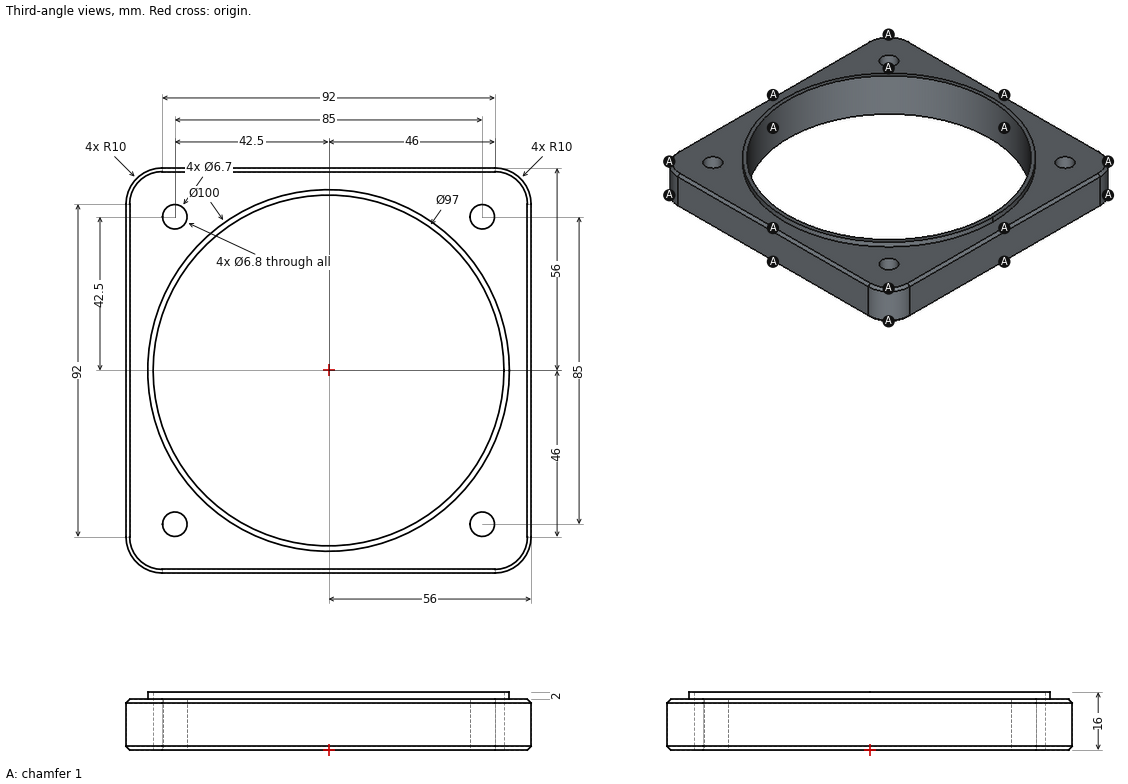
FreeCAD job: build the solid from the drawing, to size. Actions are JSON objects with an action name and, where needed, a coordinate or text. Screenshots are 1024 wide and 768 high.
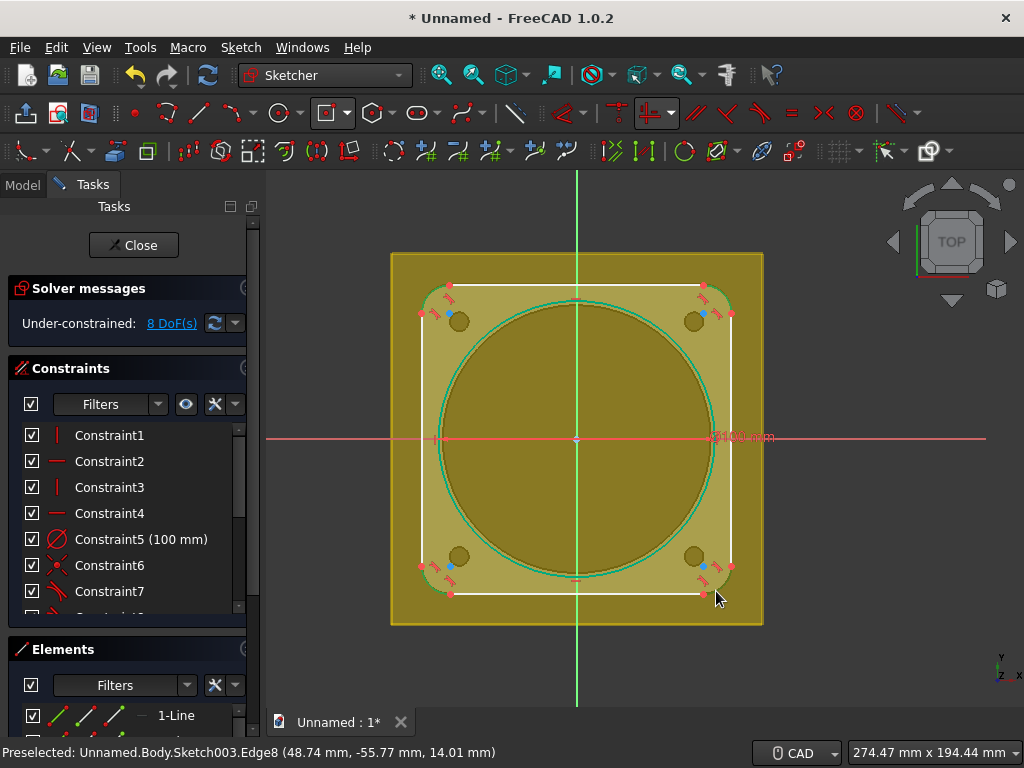
{"action": "left_click", "coordinate": [792, 114]}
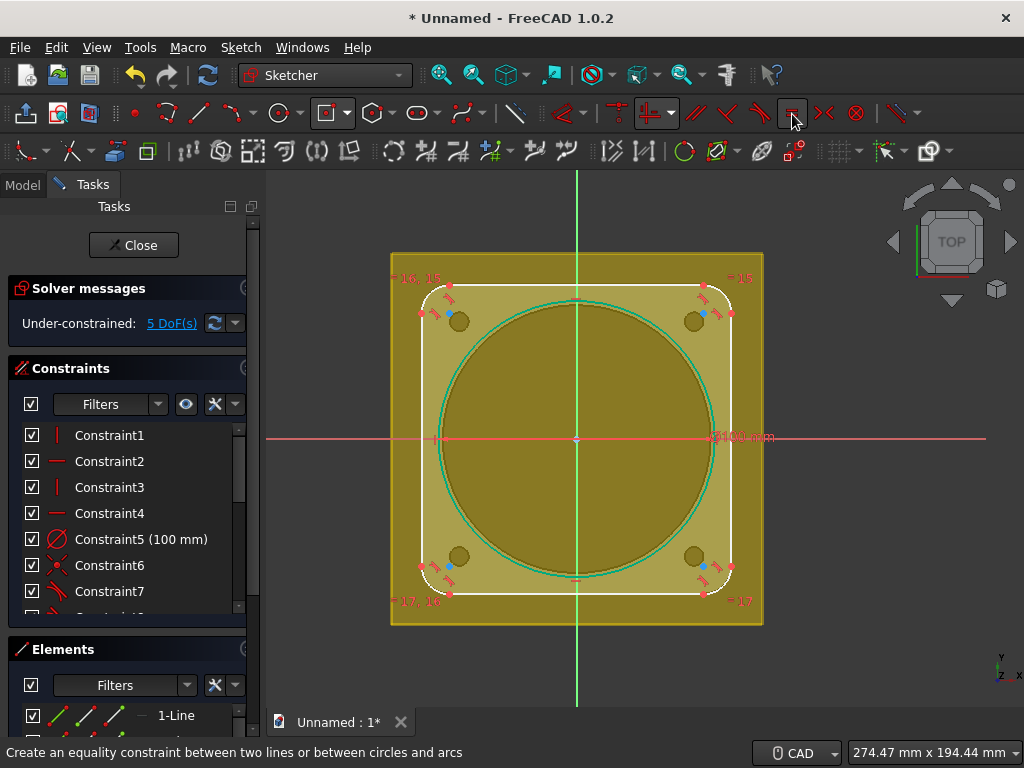
{"action": "left_click", "coordinate": [562, 114]}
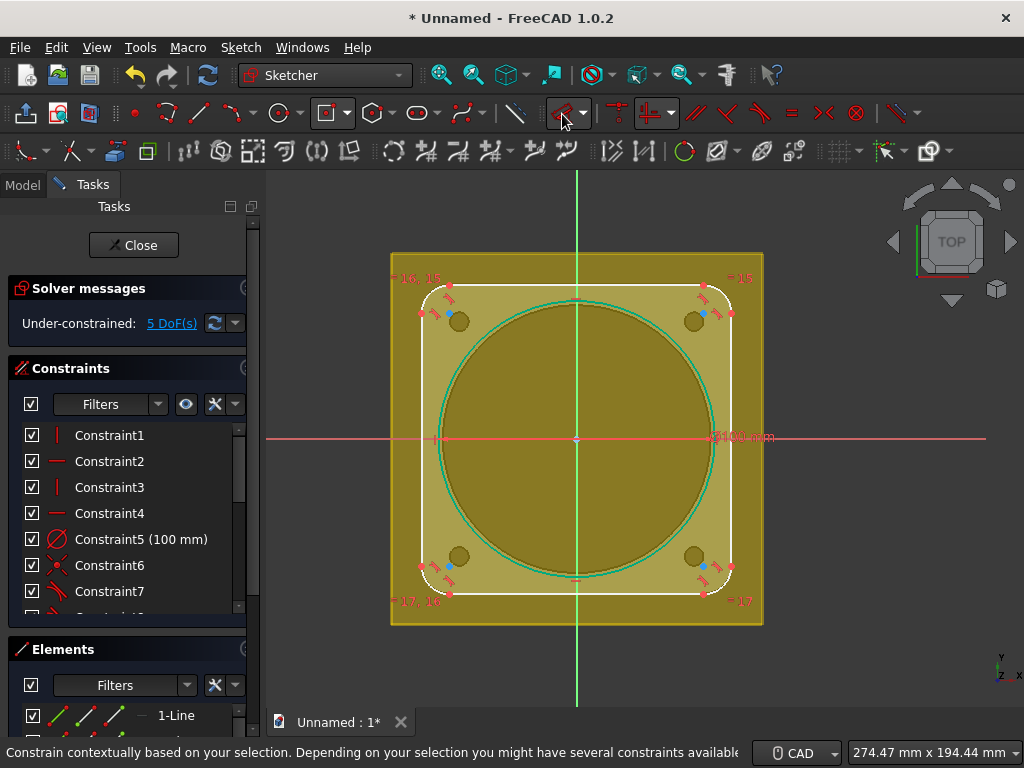
{"action": "scroll", "coordinate": [728, 301], "scroll_direction": "up", "scroll_amount": 2}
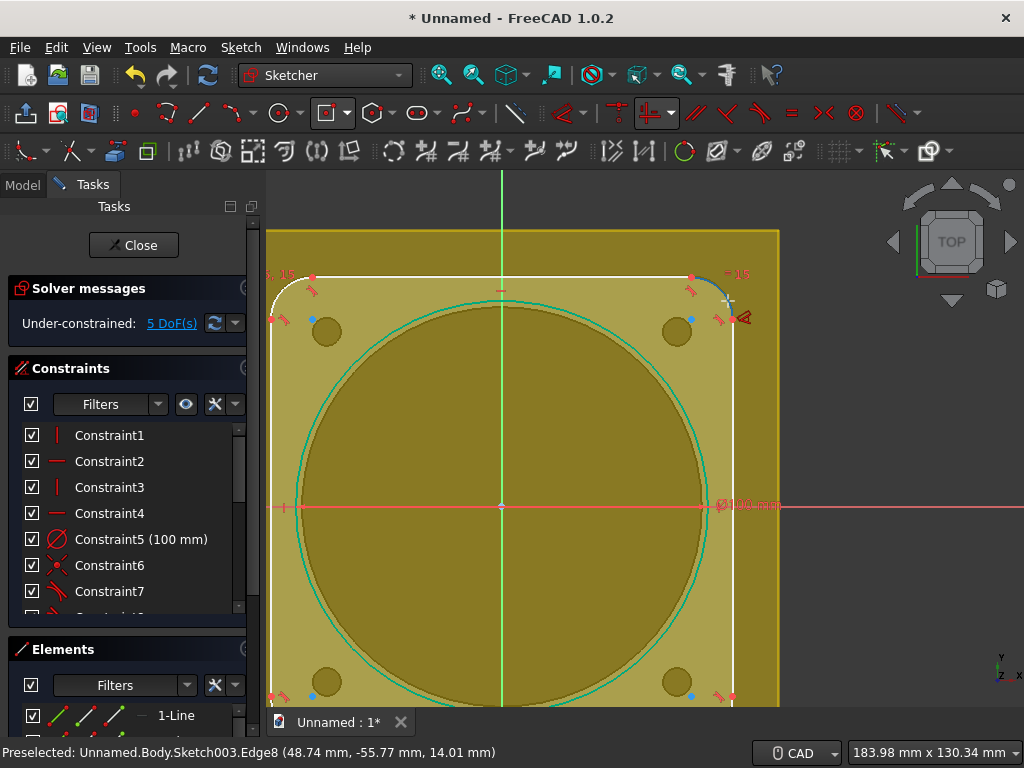
{"action": "left_click", "coordinate": [728, 300]}
{"action": "left_click", "coordinate": [756, 285]}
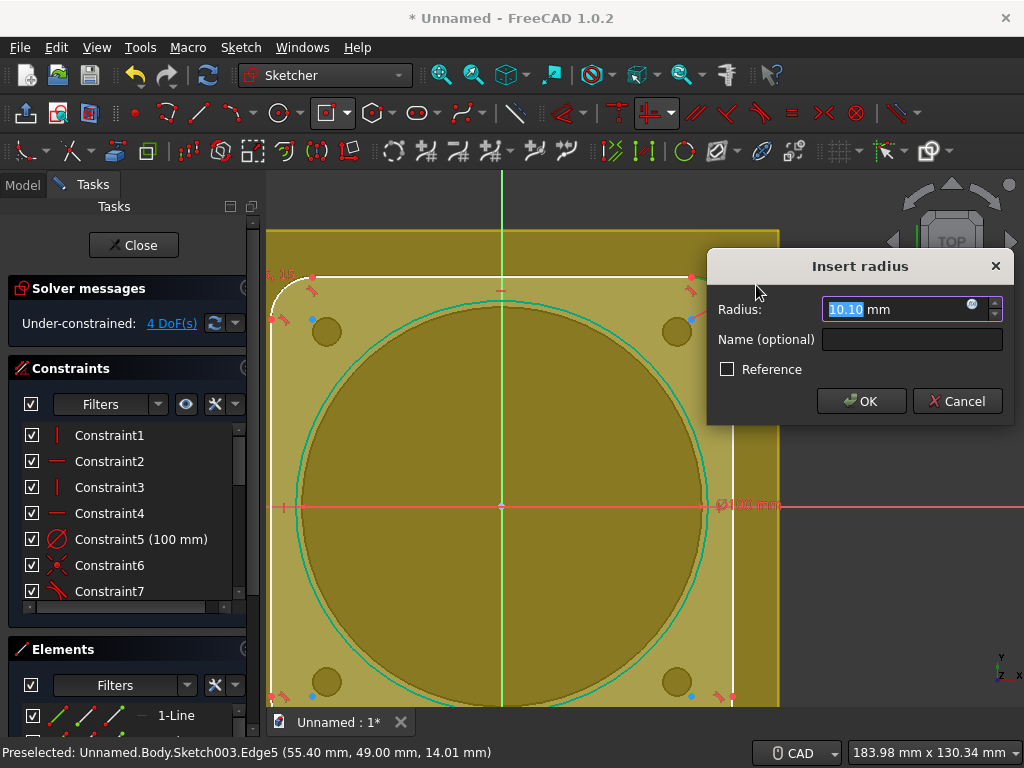
{"action": "type", "text": "10"}
{"action": "key", "text": "Return"}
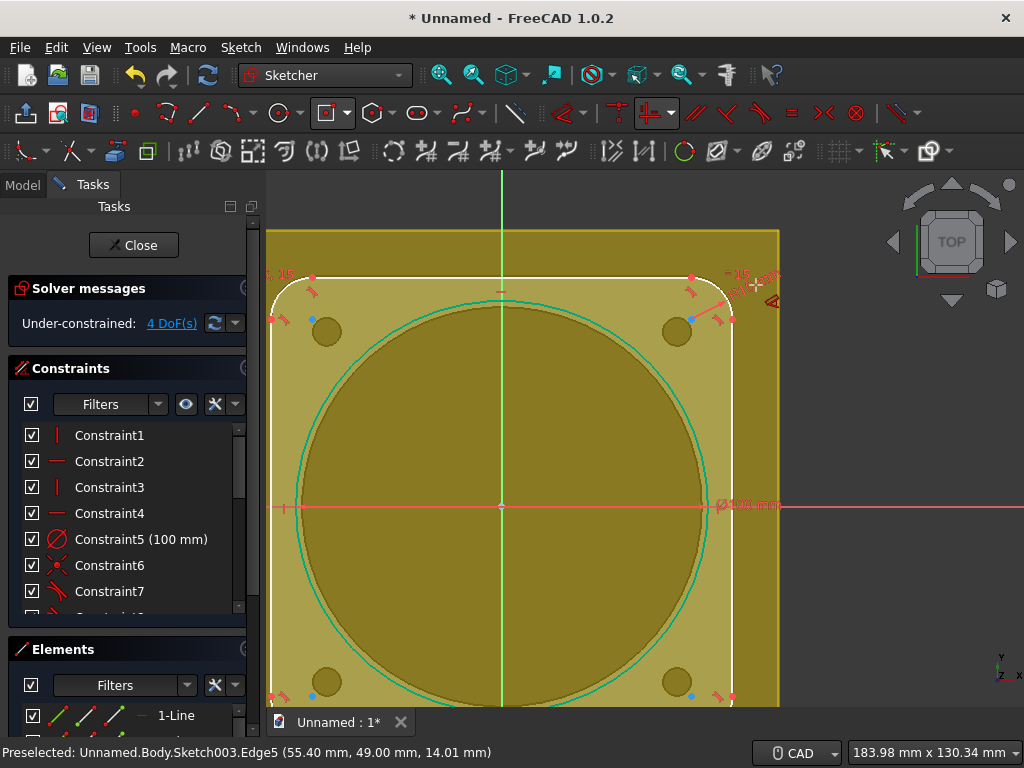
{"action": "left_click", "coordinate": [732, 584]}
{"action": "left_click", "coordinate": [766, 416]}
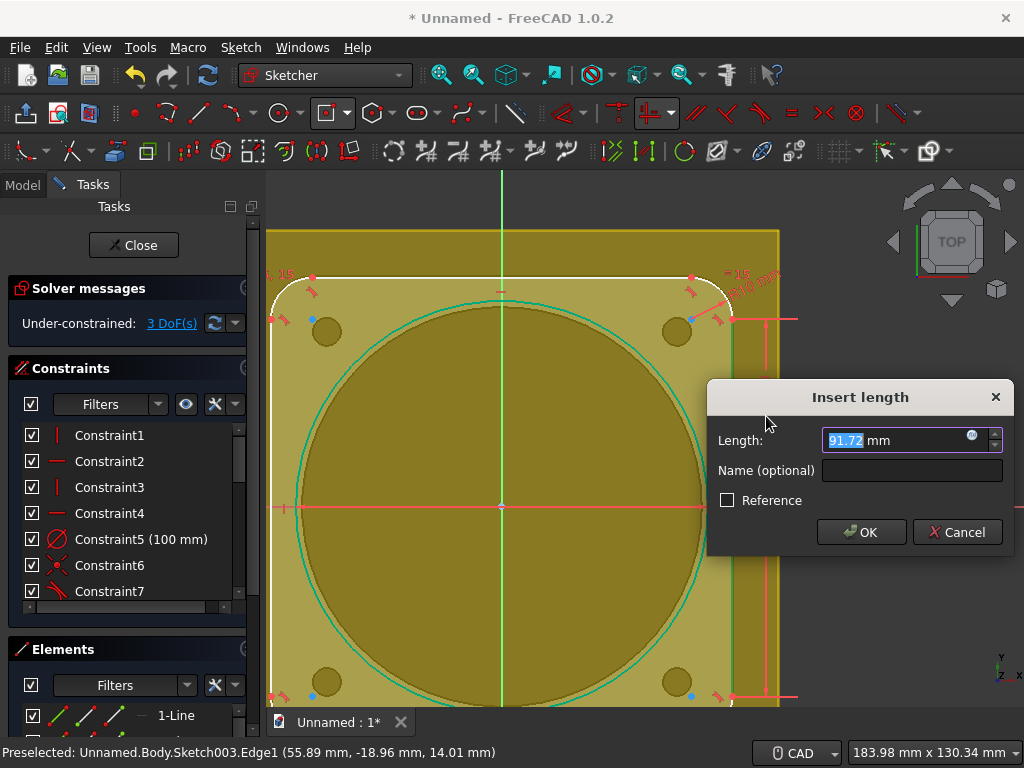
{"action": "type", "text": "92"}
{"action": "key", "text": "Return"}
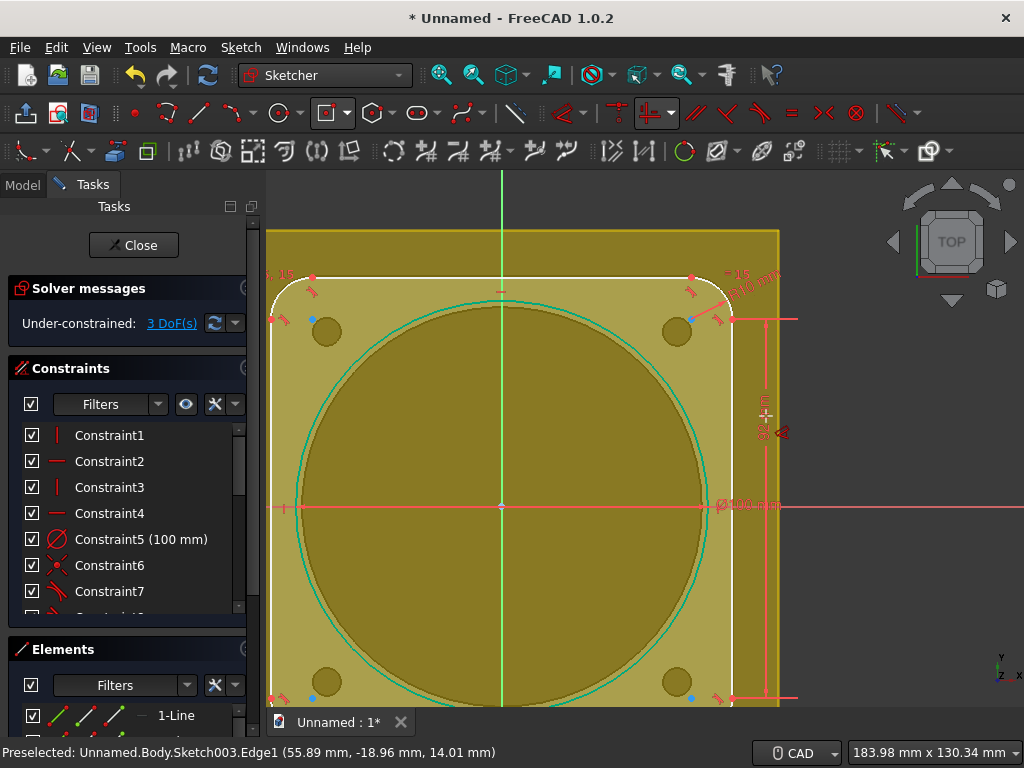
{"action": "left_click", "coordinate": [577, 278]}
{"action": "left_click", "coordinate": [415, 244]}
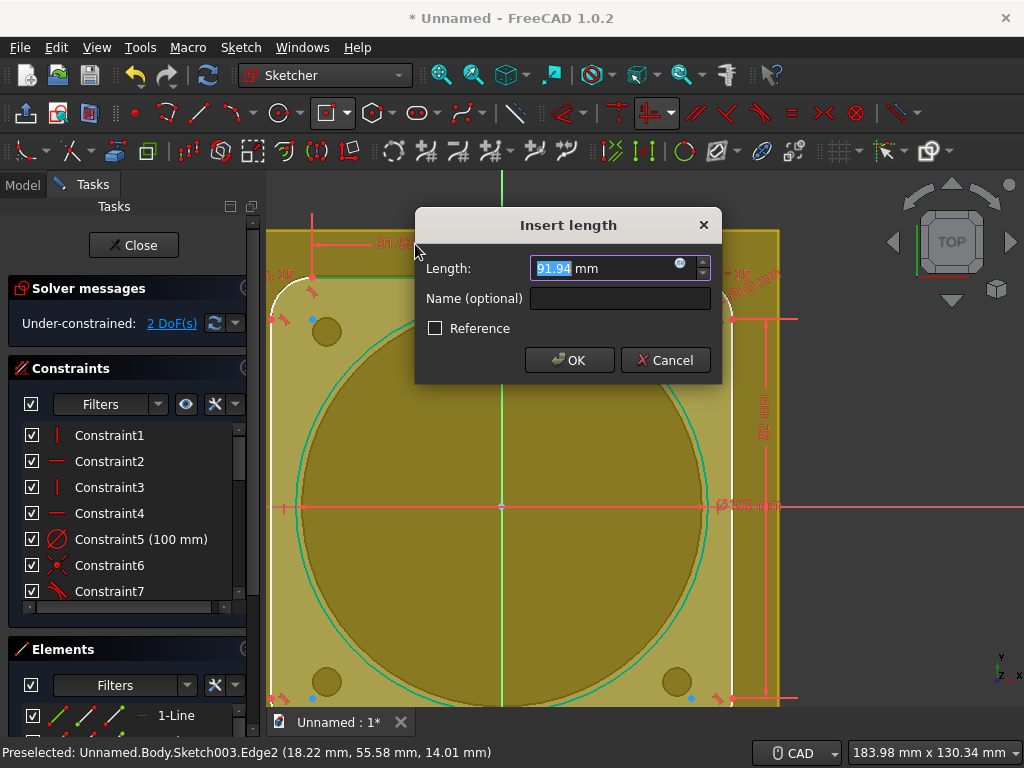
{"action": "type", "text": "92"}
{"action": "key", "text": "Return"}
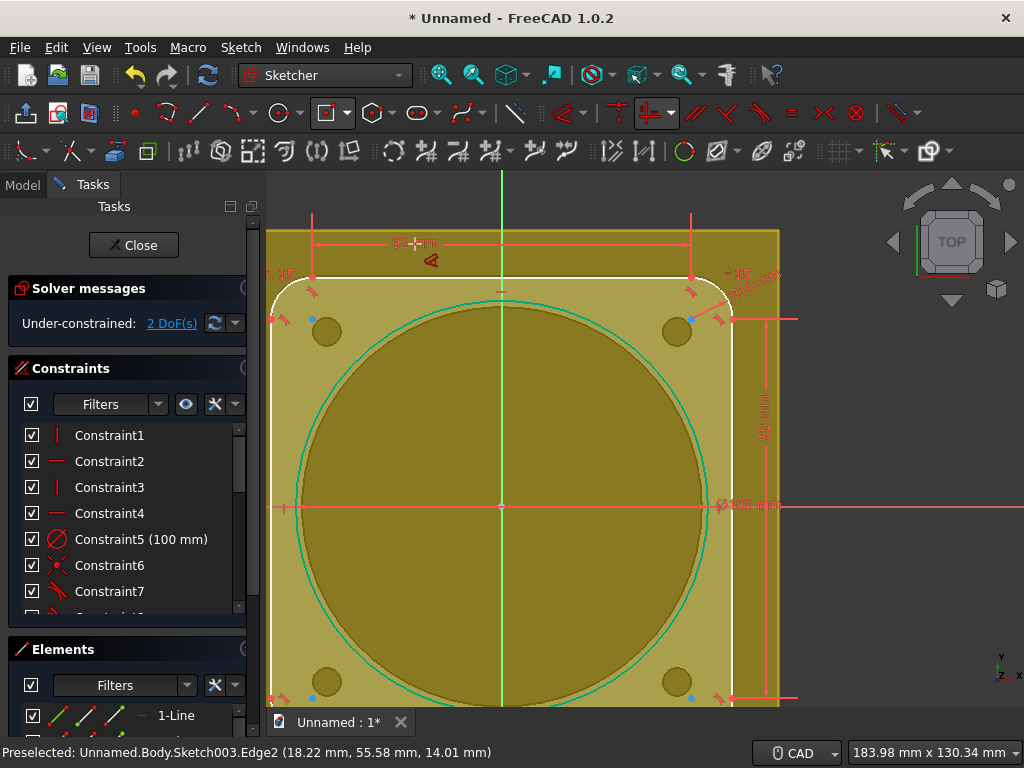
{"action": "scroll", "coordinate": [728, 299], "scroll_direction": "down", "scroll_amount": 2}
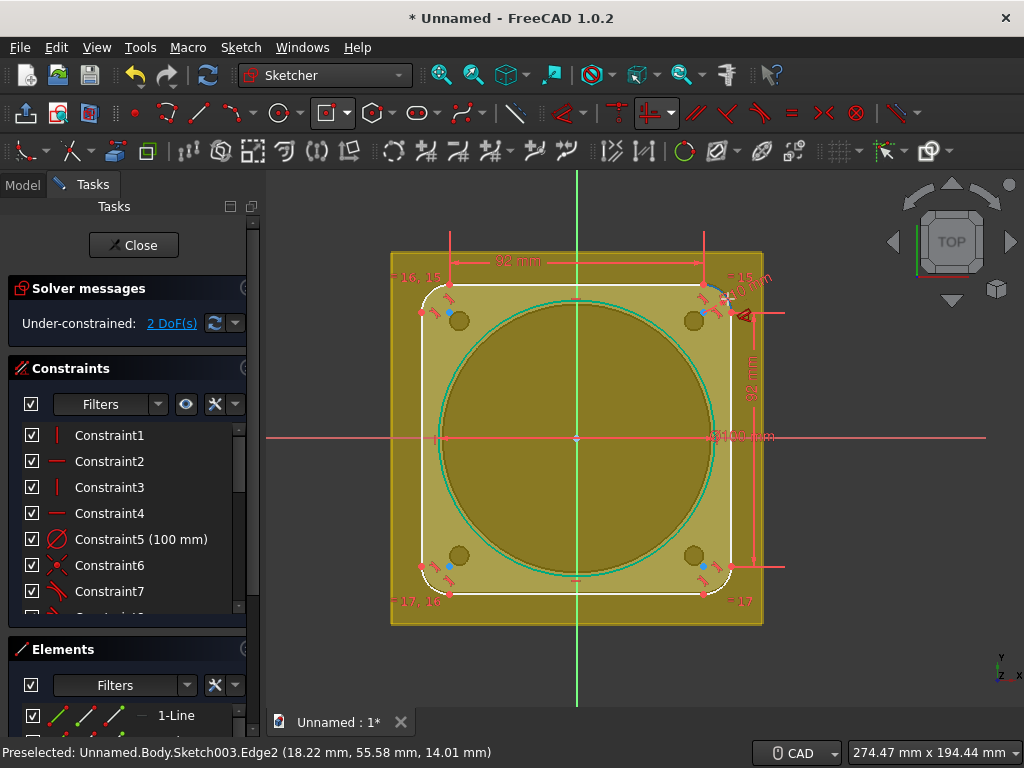
{"action": "left_click", "coordinate": [731, 567]}
{"action": "left_click", "coordinate": [654, 404]}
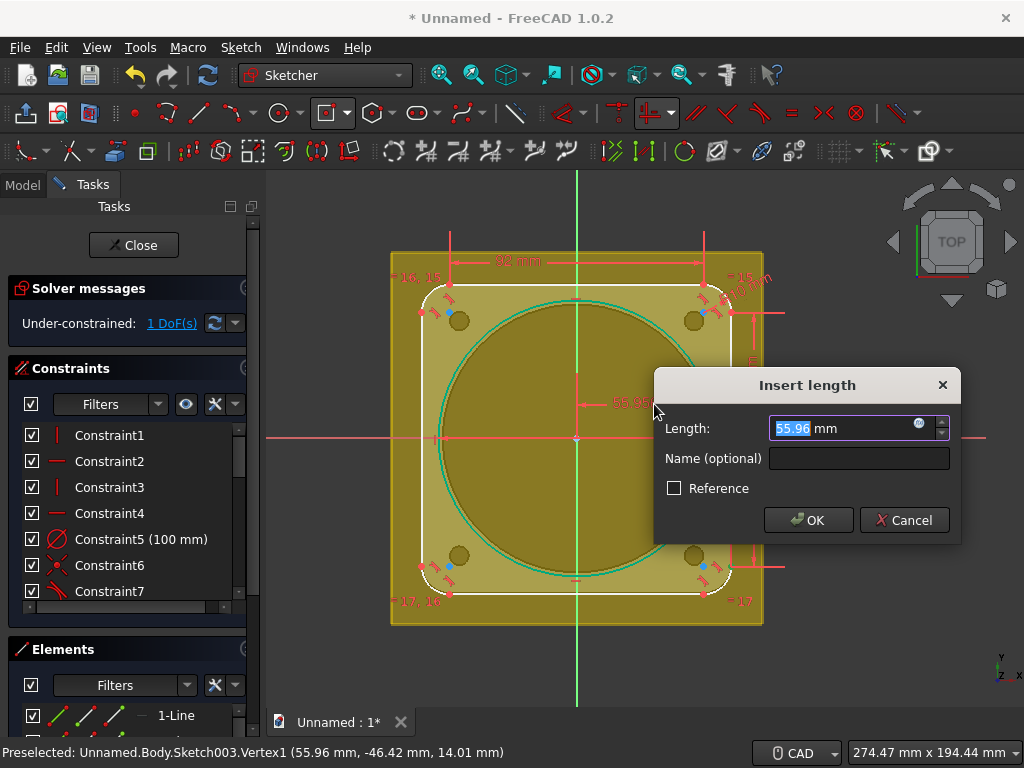
{"action": "type", "text": "56"}
{"action": "key", "text": "Return"}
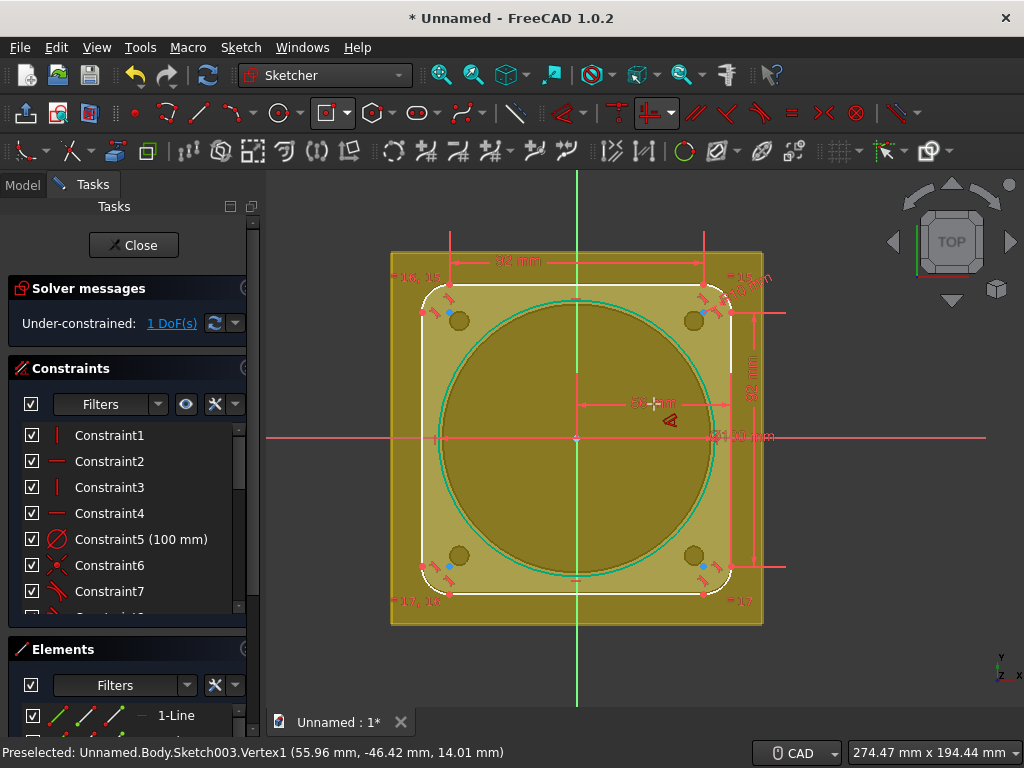
{"action": "left_click", "coordinate": [731, 567]}
{"action": "left_click", "coordinate": [765, 503]}